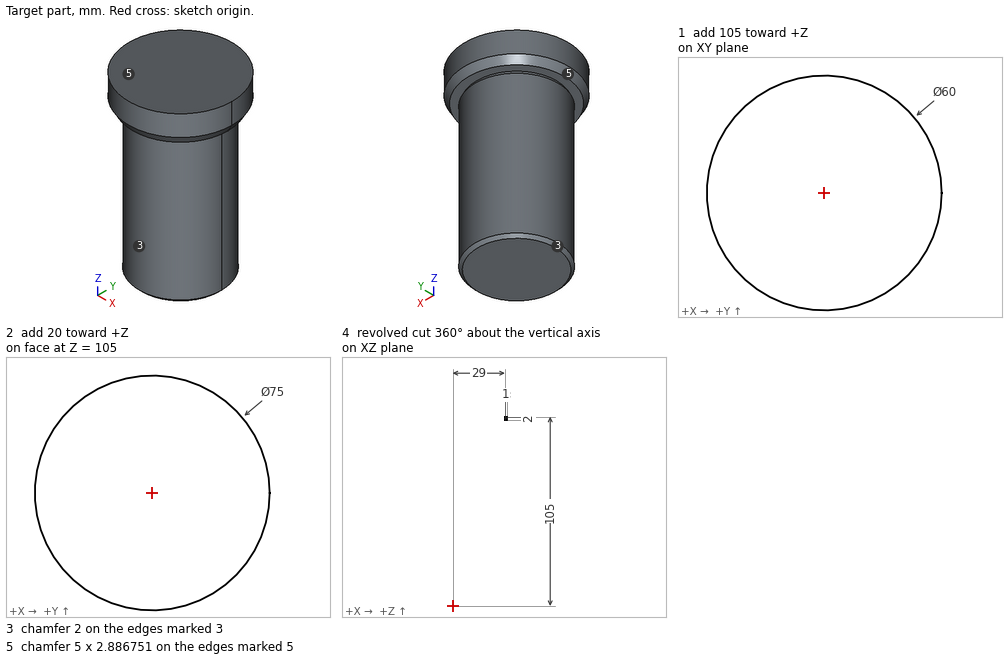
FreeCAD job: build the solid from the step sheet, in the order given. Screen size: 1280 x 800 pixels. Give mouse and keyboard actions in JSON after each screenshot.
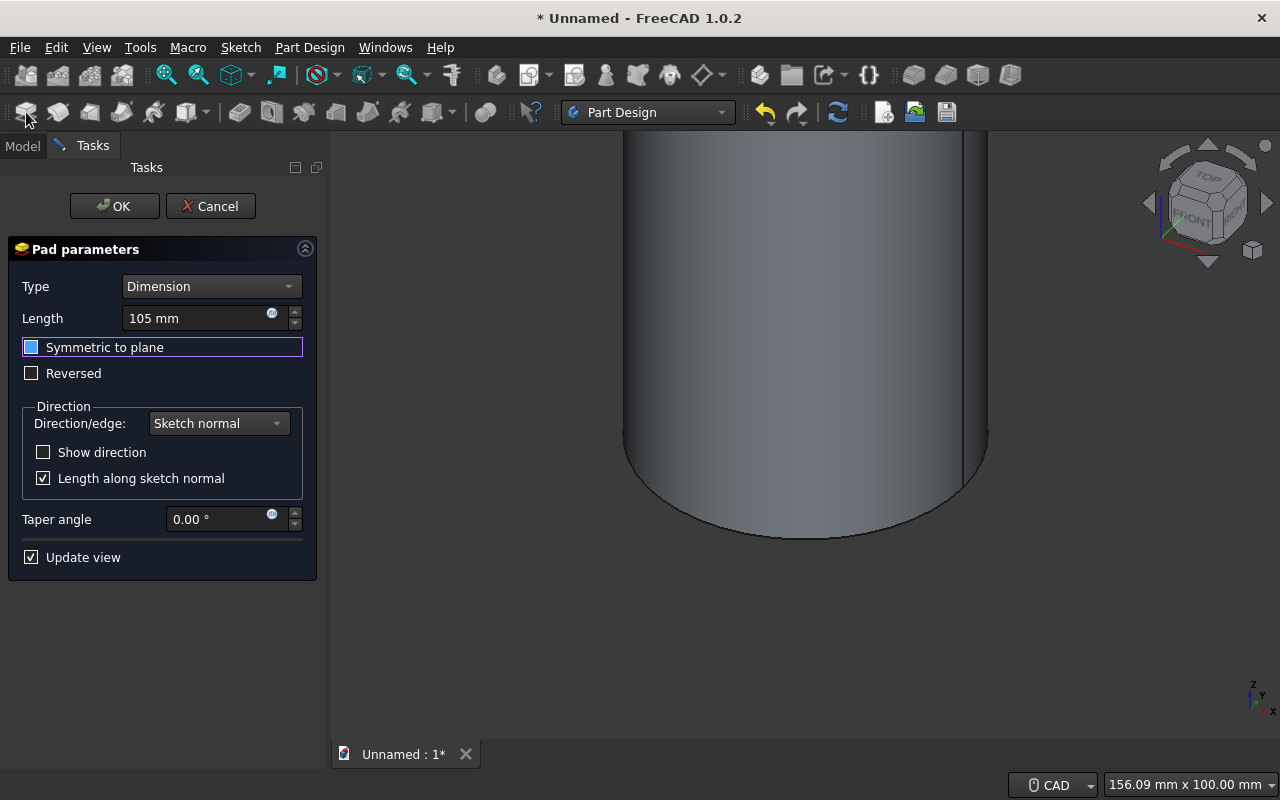
{"action": "left_click", "coordinate": [115, 206]}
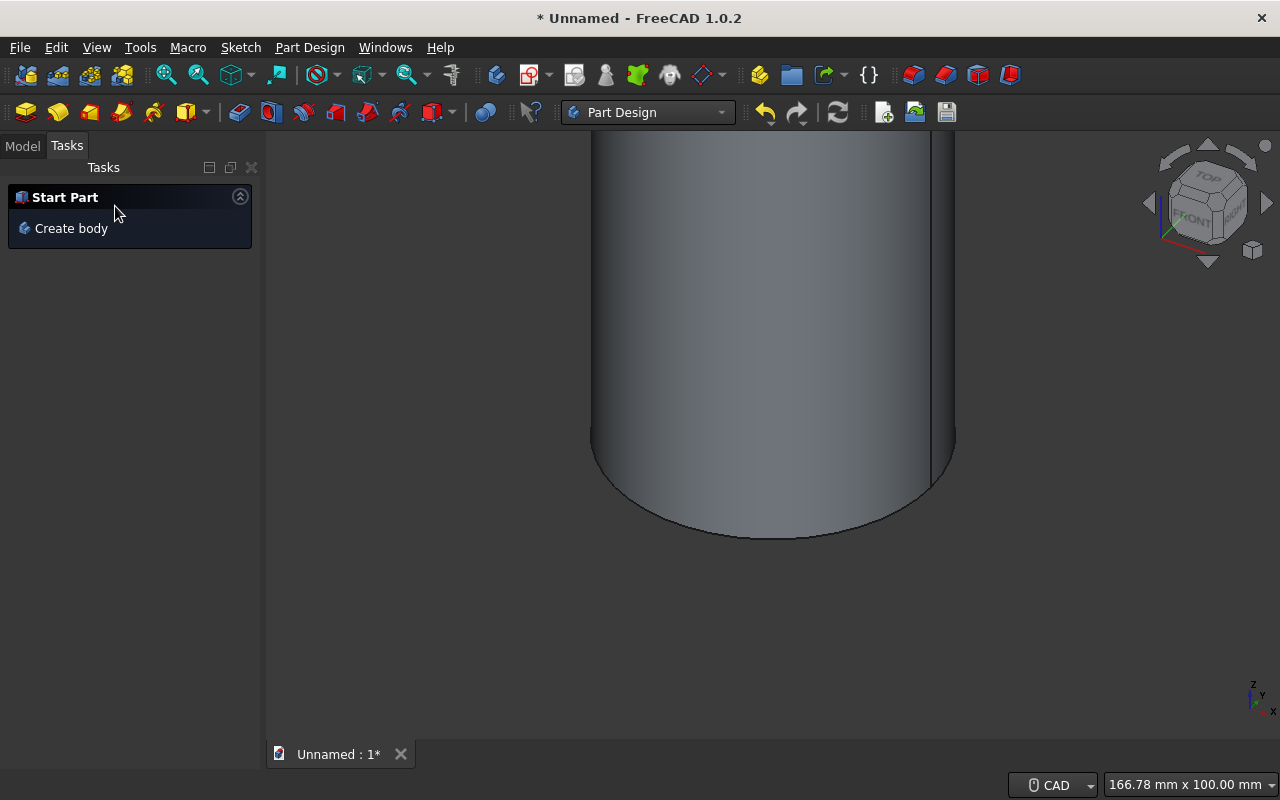
{"action": "left_click", "coordinate": [168, 76]}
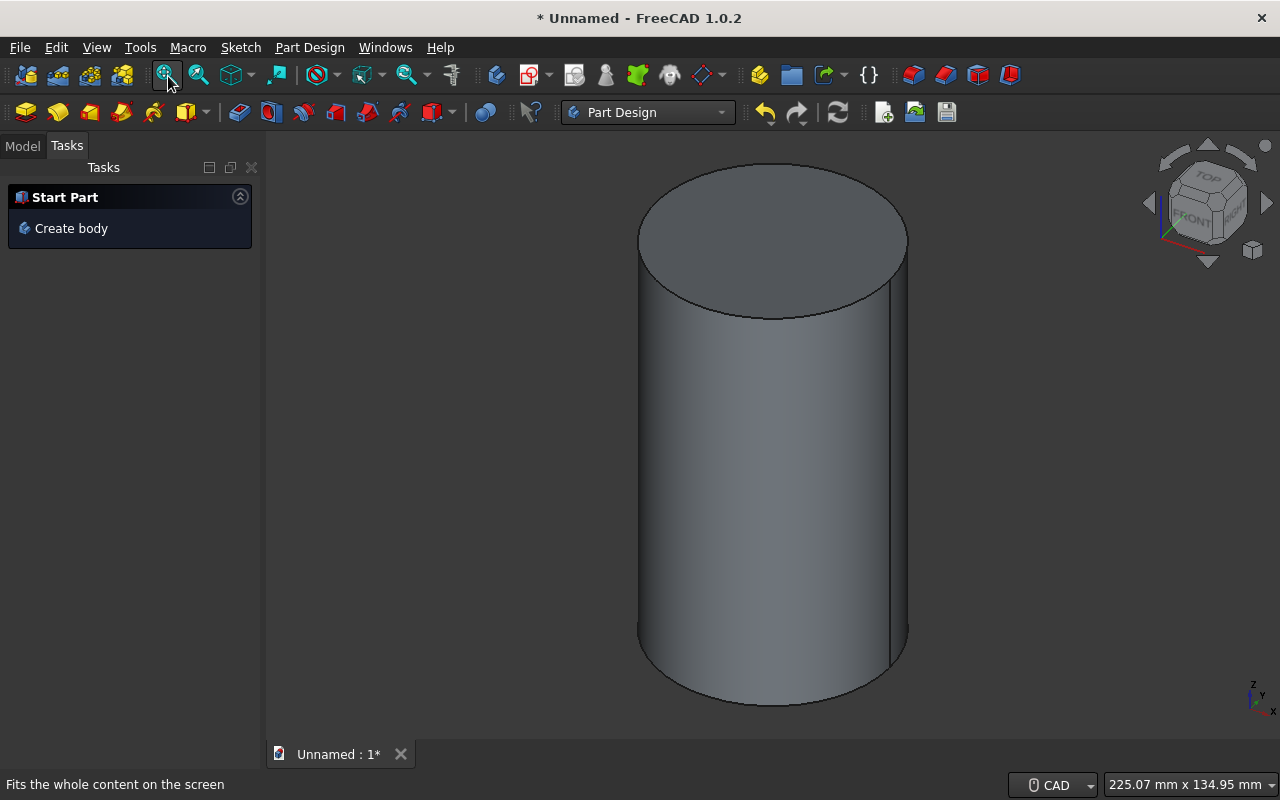
{"action": "left_click", "coordinate": [773, 240]}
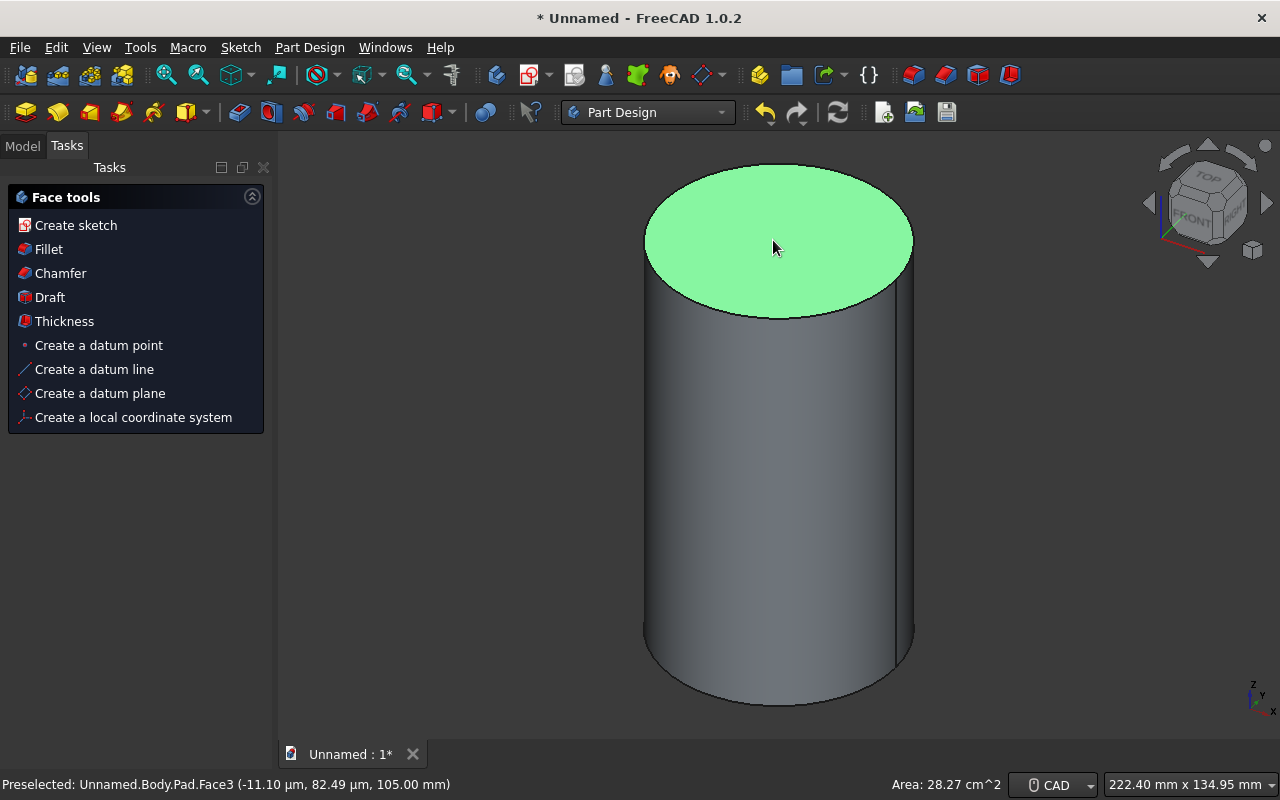
{"action": "left_click", "coordinate": [530, 76]}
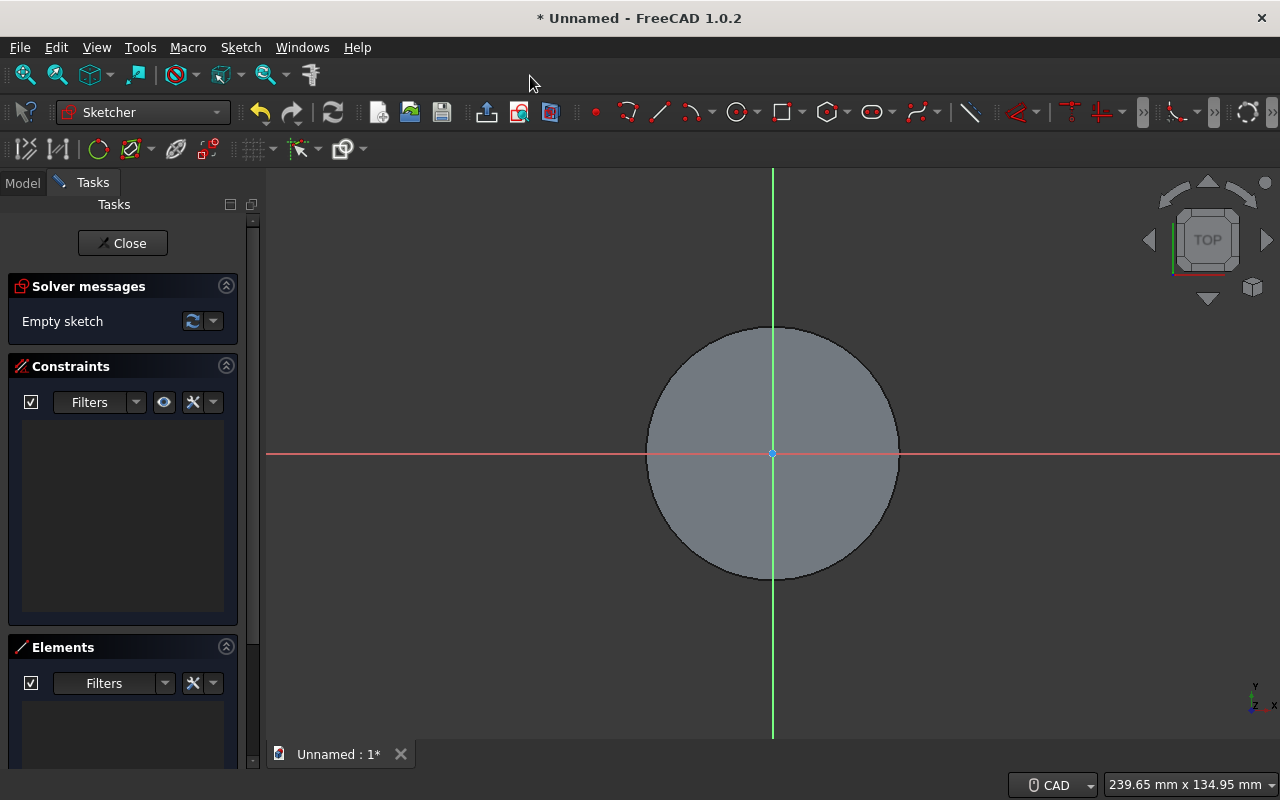
{"action": "left_click", "coordinate": [738, 112]}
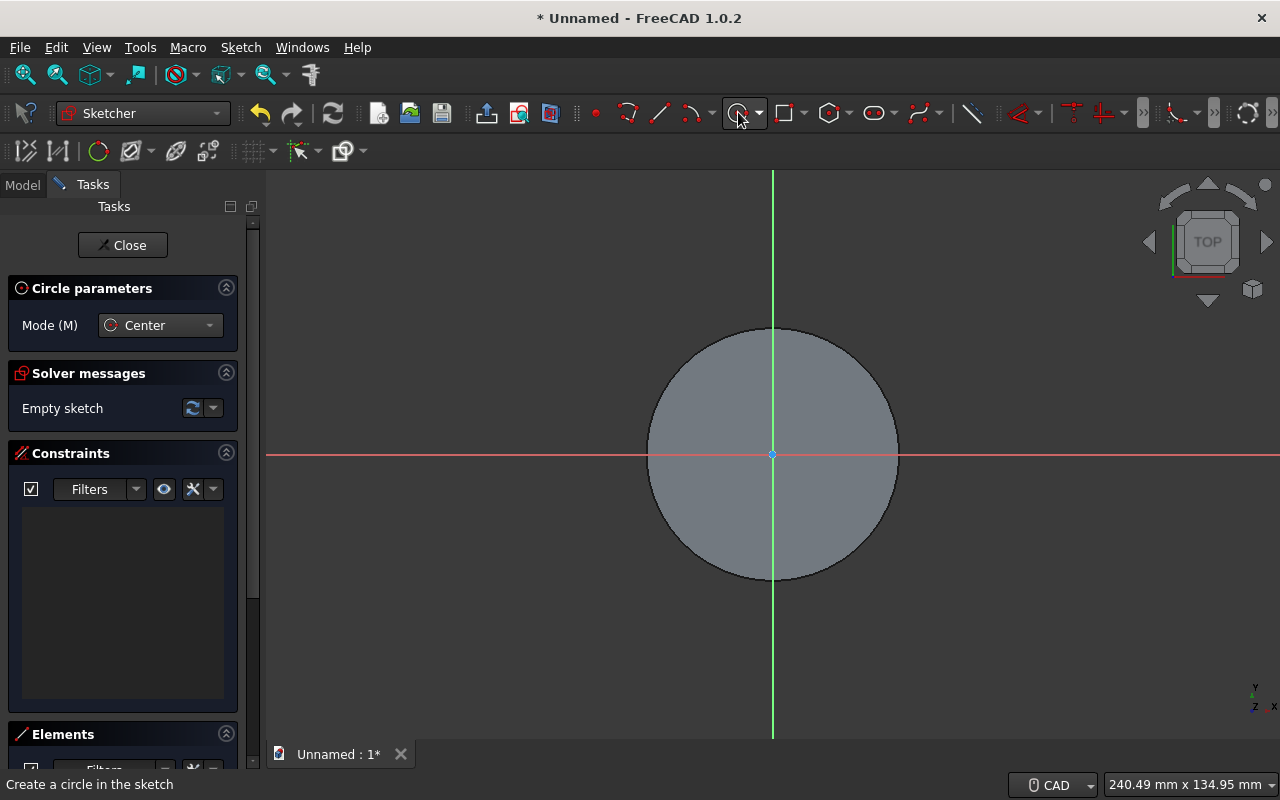
{"action": "left_click", "coordinate": [773, 454]}
{"action": "mouse_move", "coordinate": [885, 343]}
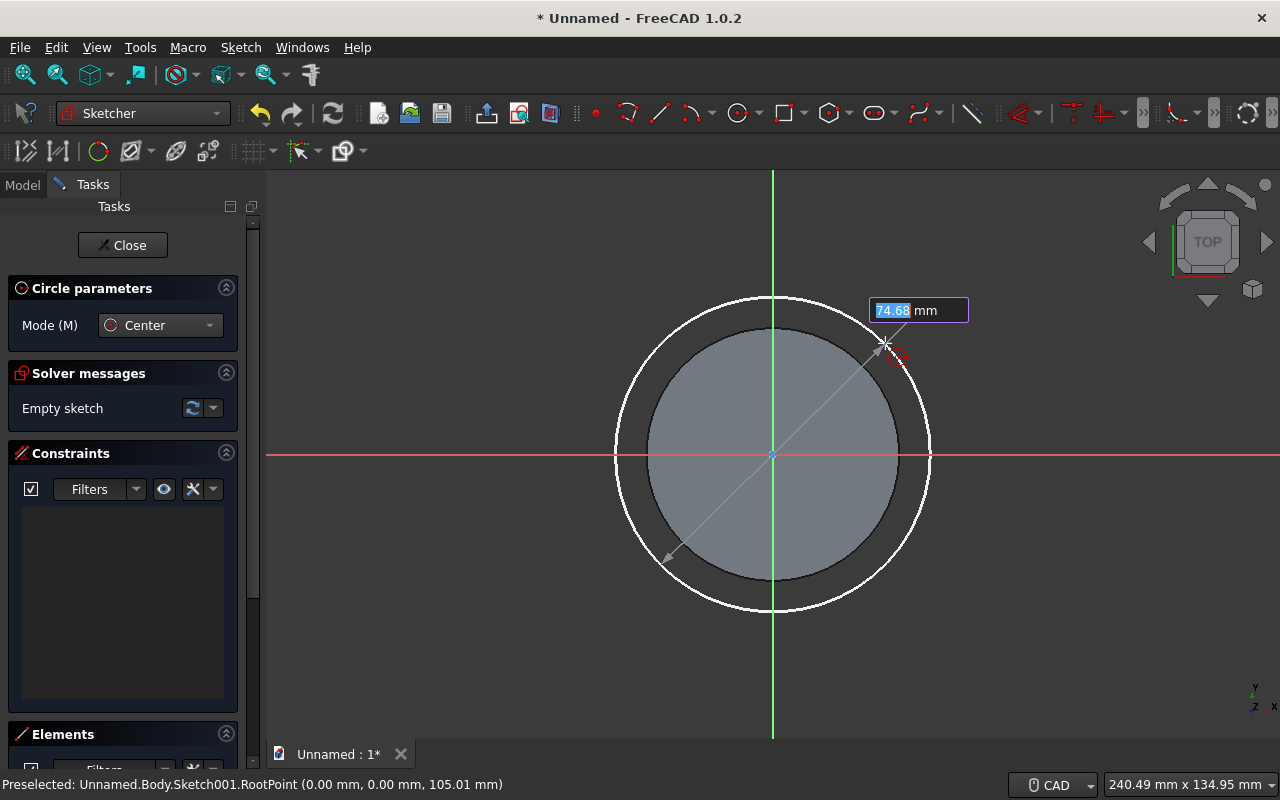
{"action": "type", "text": "75"}
{"action": "key", "text": "Return"}
{"action": "key", "text": "Escape"}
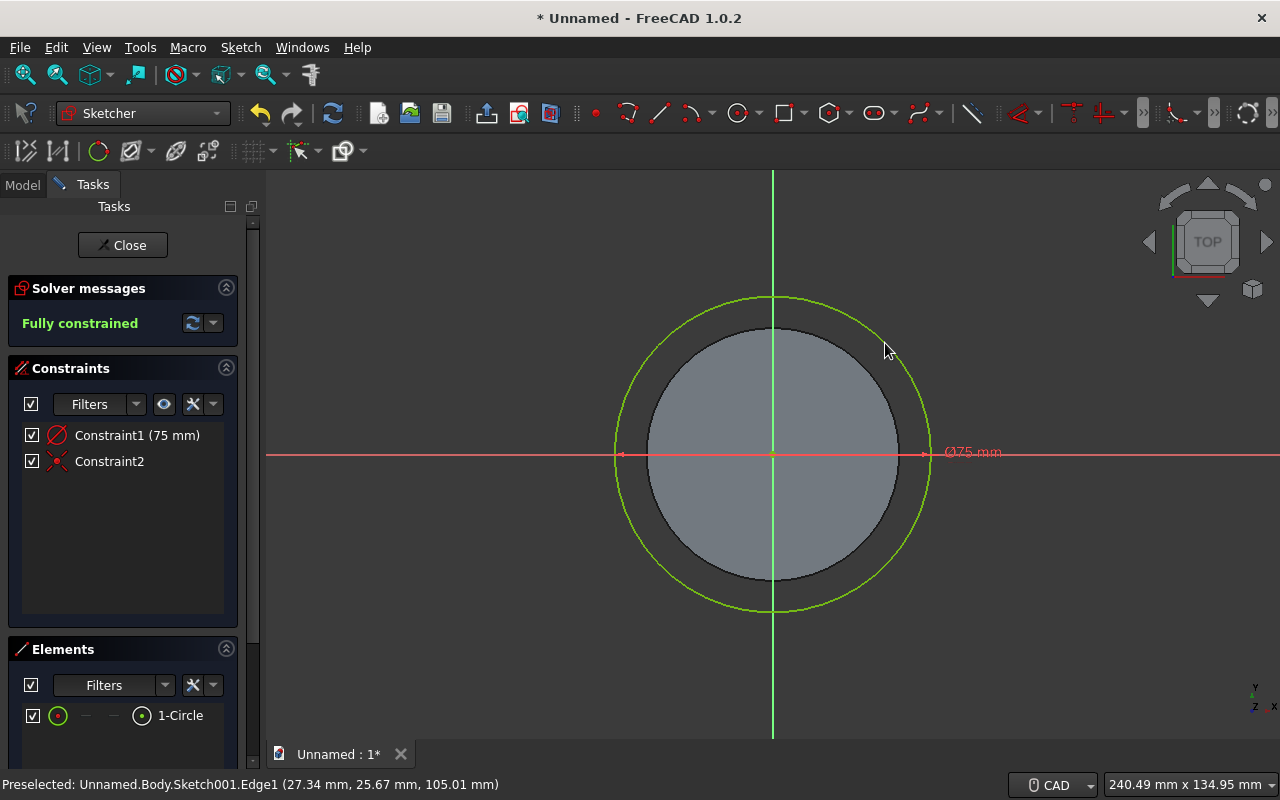
{"action": "left_click", "coordinate": [123, 245]}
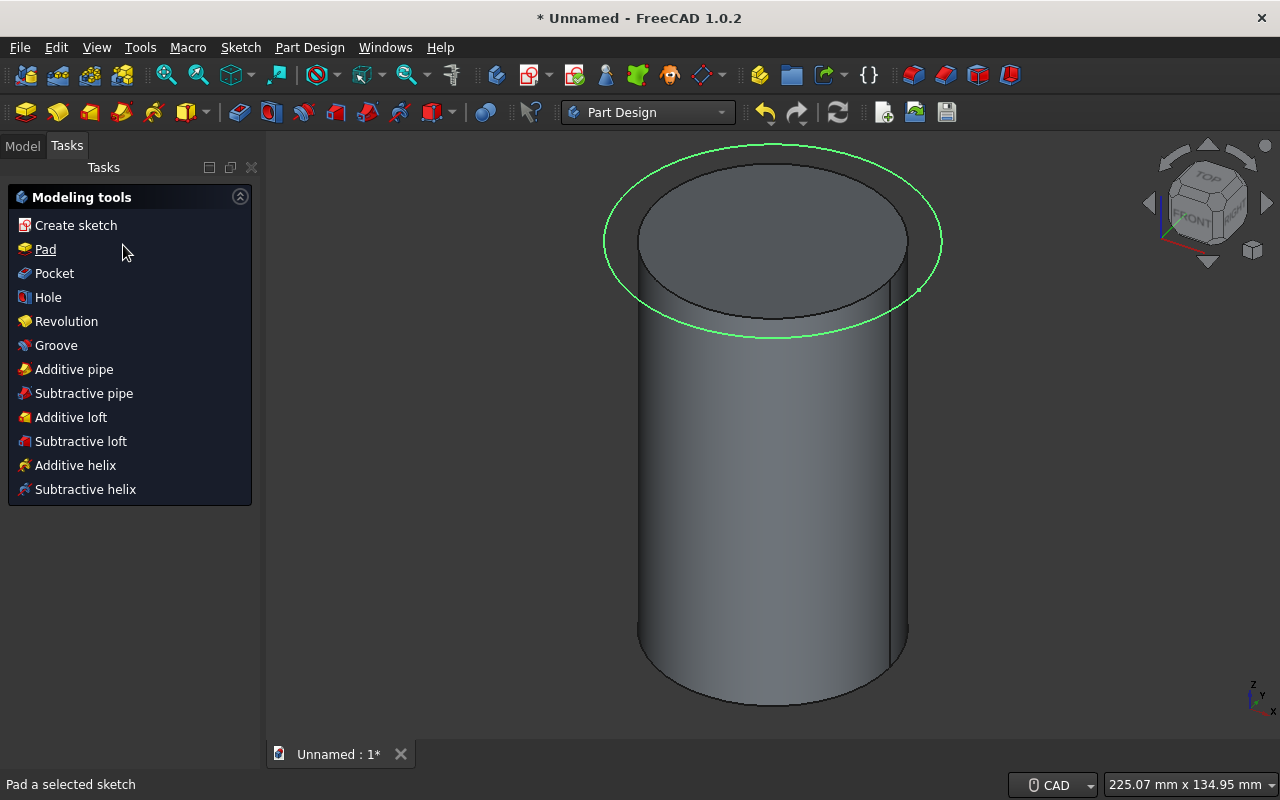
{"action": "left_click", "coordinate": [26, 112]}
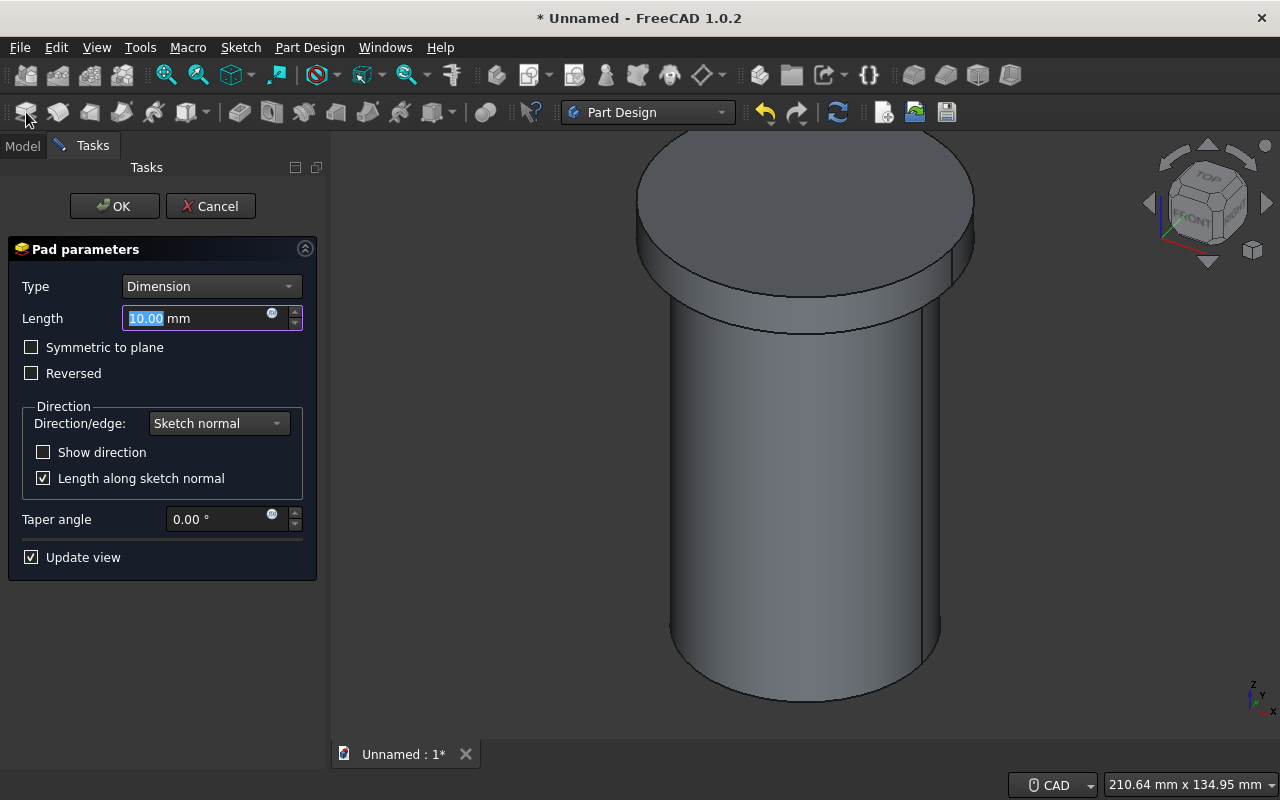
{"action": "type", "text": "20"}
{"action": "key", "text": "Tab"}